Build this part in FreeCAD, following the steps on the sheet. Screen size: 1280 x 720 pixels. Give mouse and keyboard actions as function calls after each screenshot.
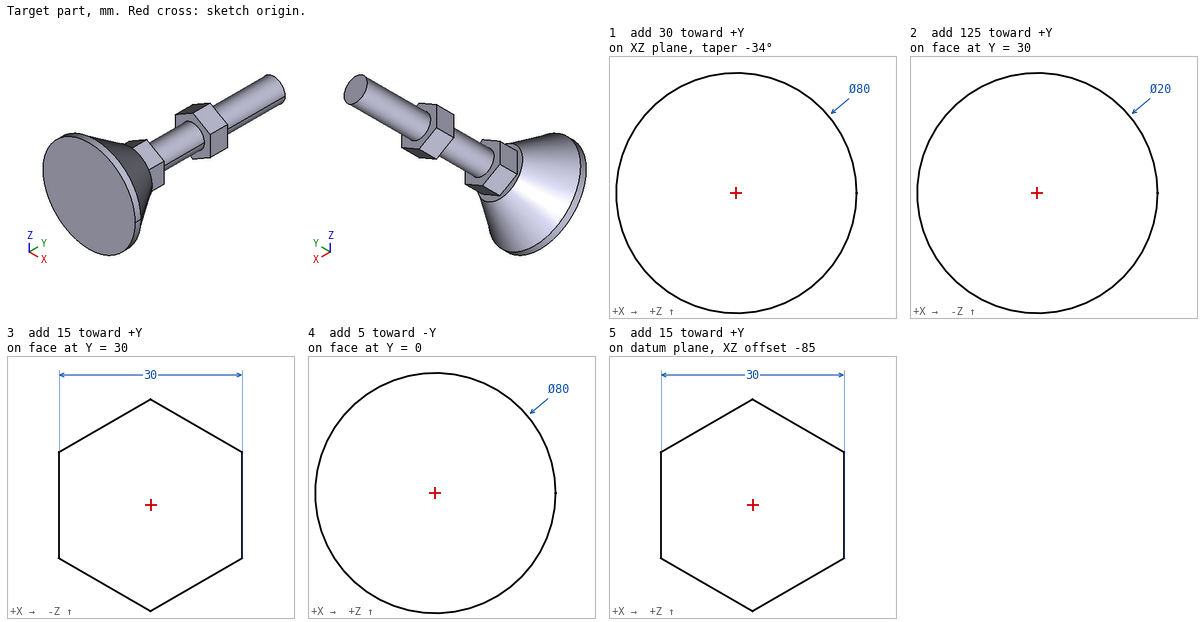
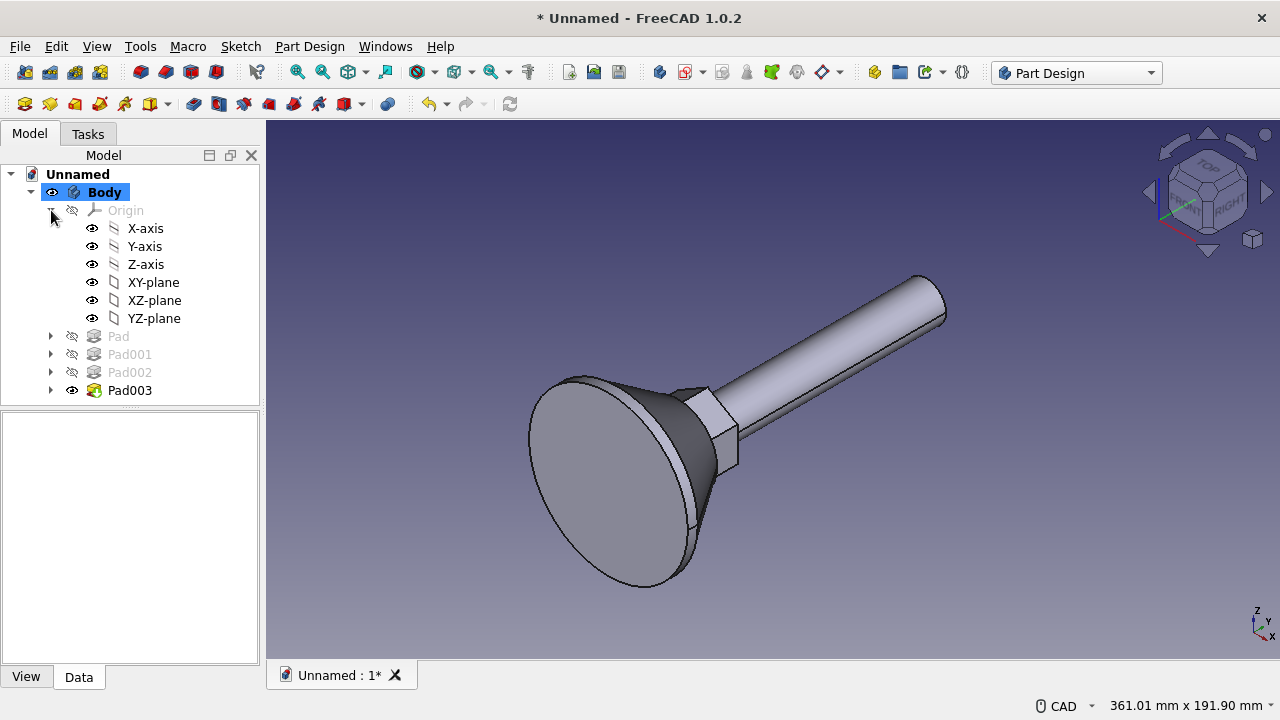
click(137, 300)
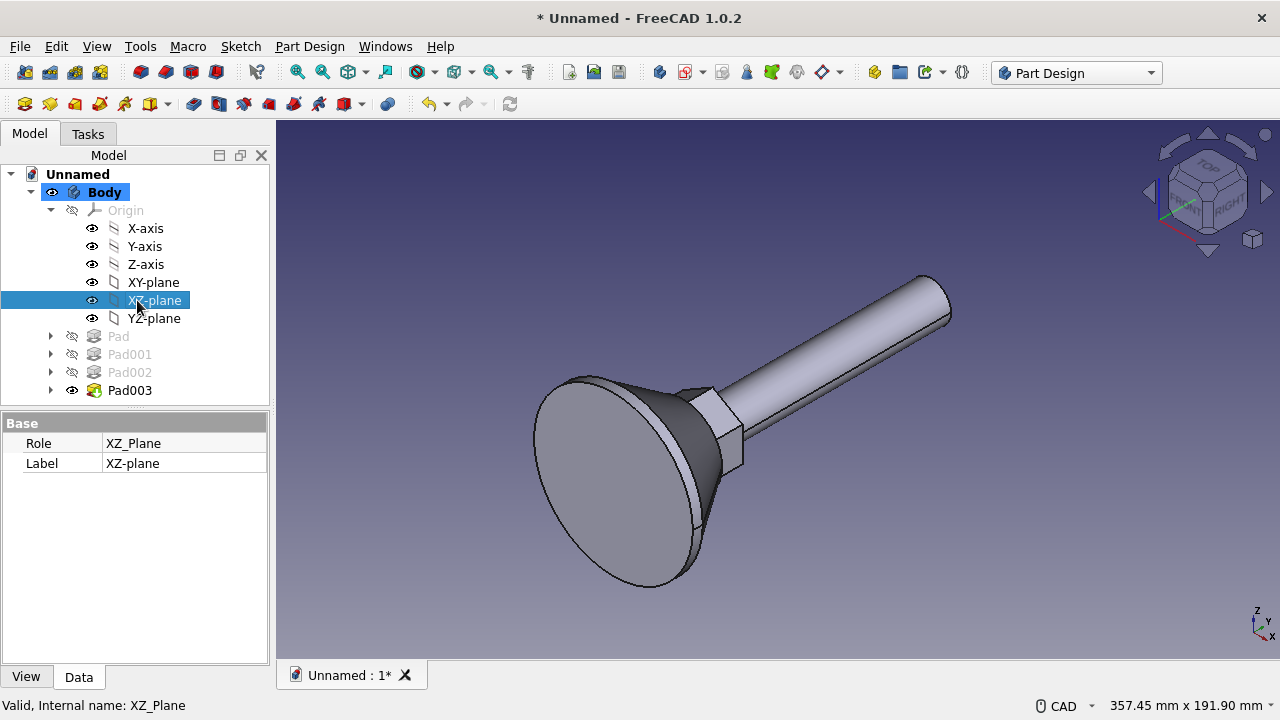
click(822, 72)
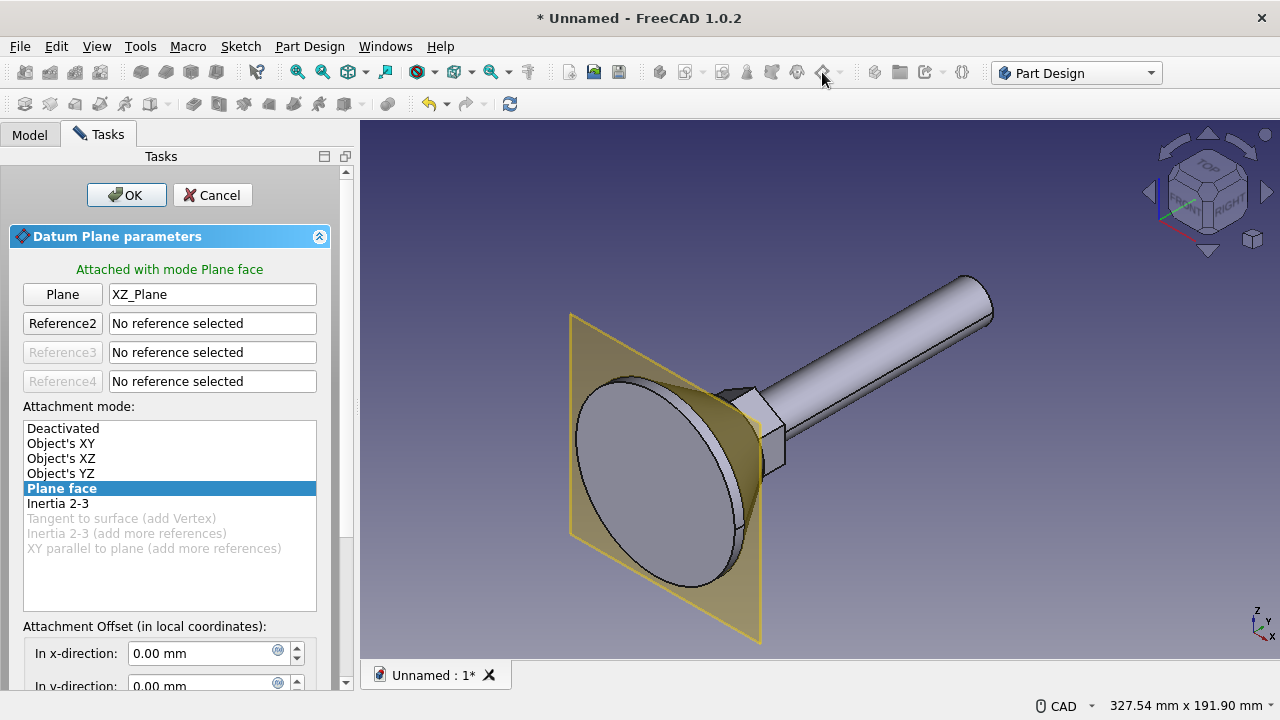
scroll(346, 428, down, 2)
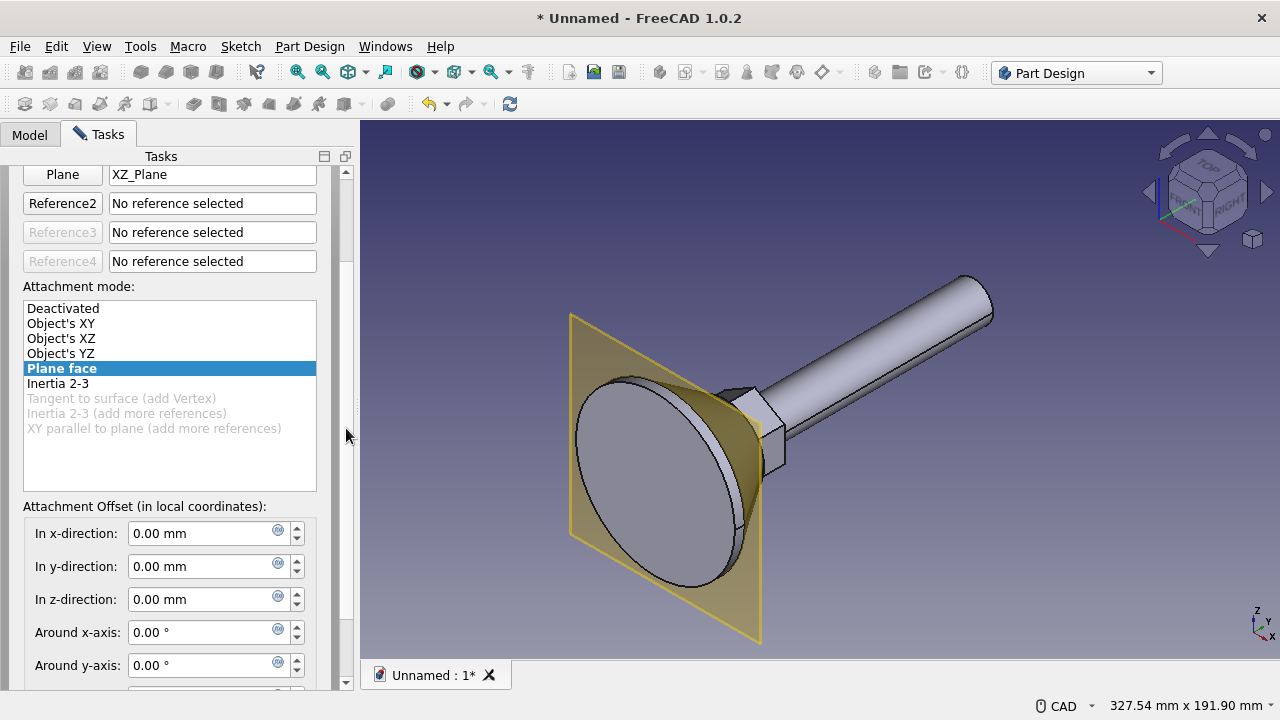
triple_click(210, 600)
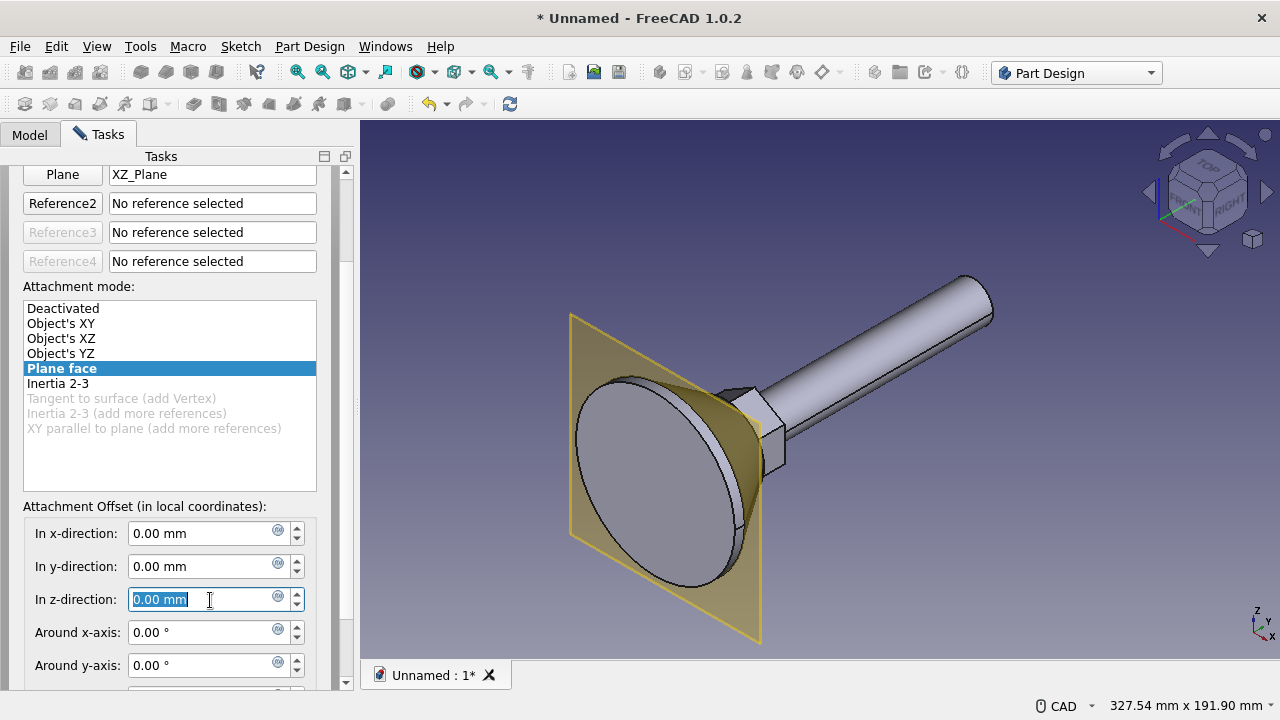
text(-85)
key(Tab)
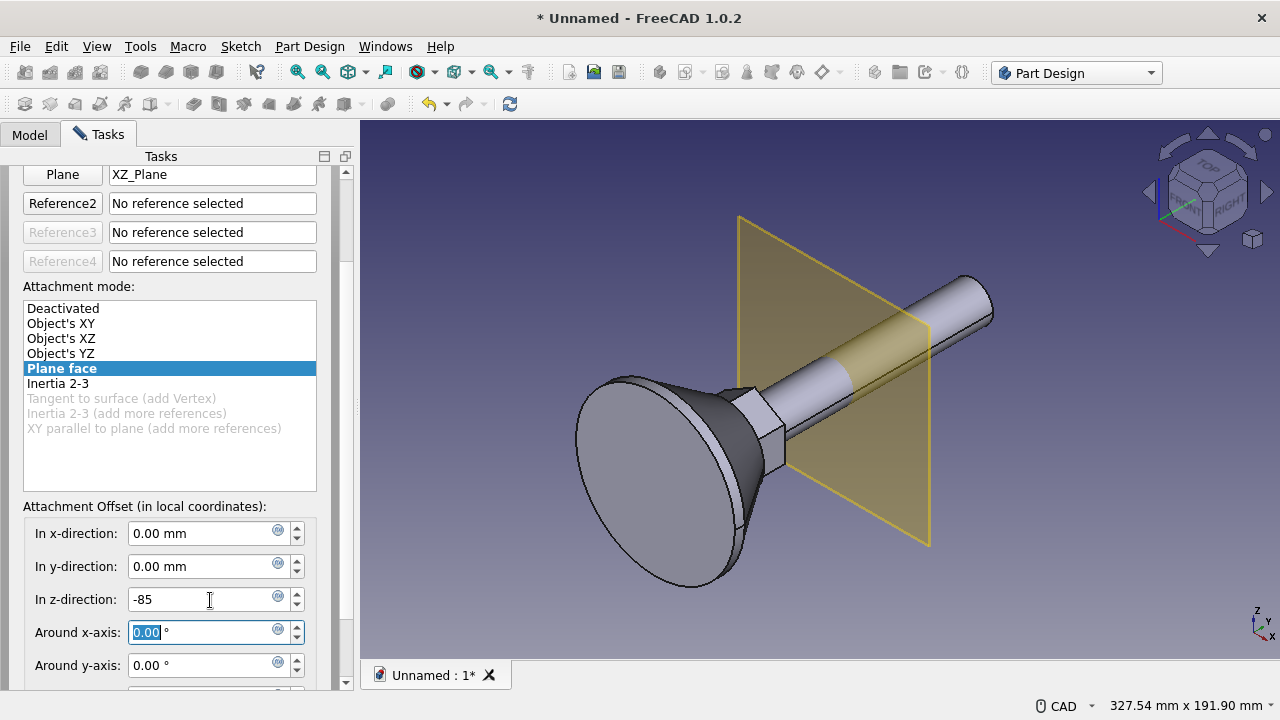
scroll(346, 428, up, 3)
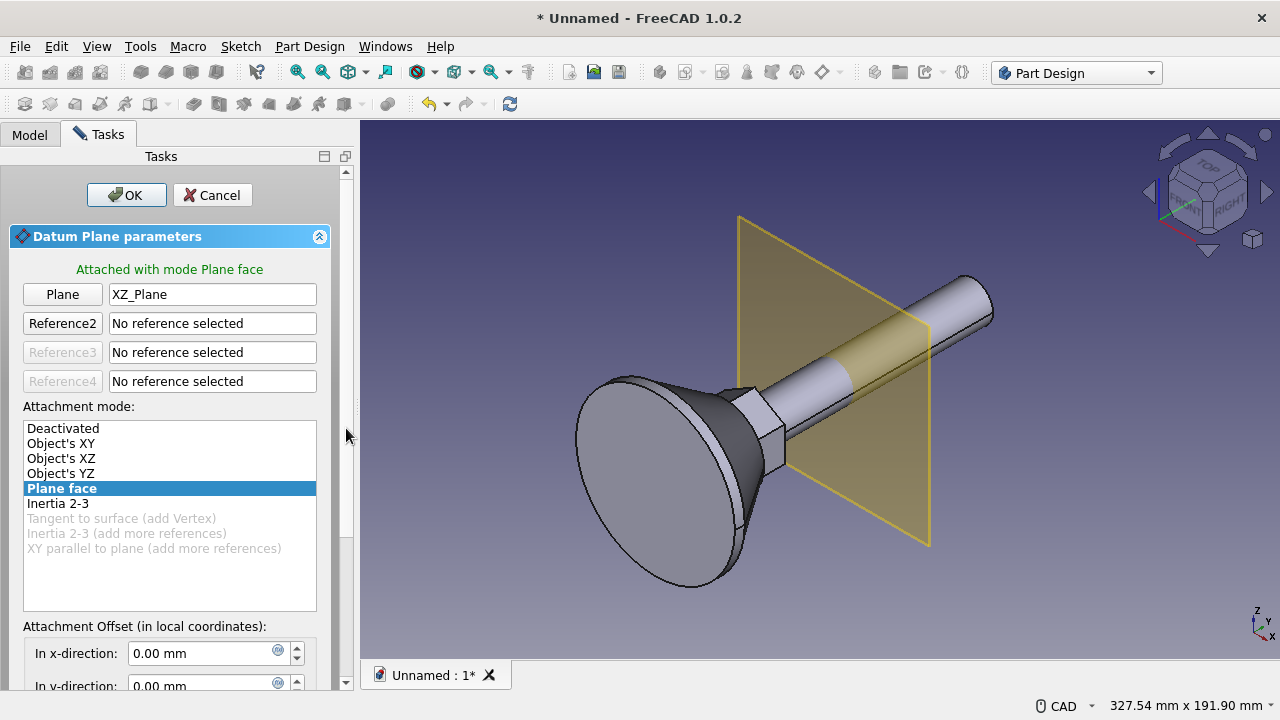
click(127, 195)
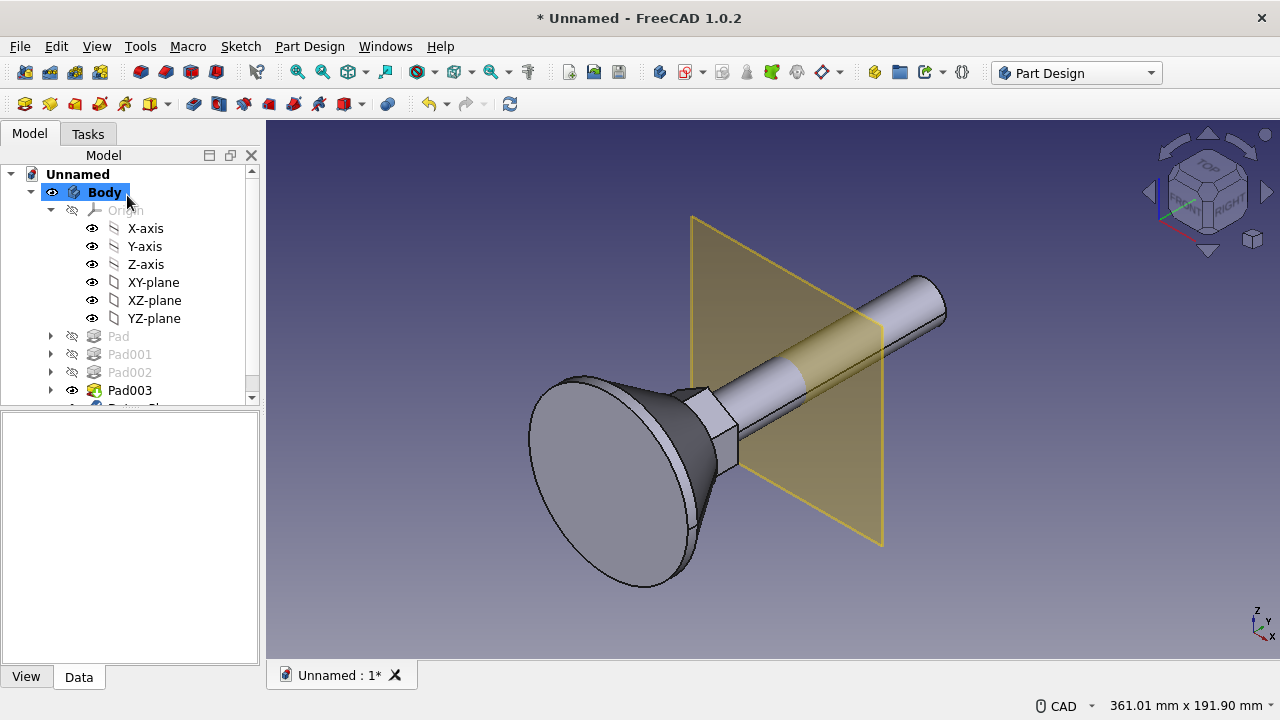
scroll(101, 278, down, 3)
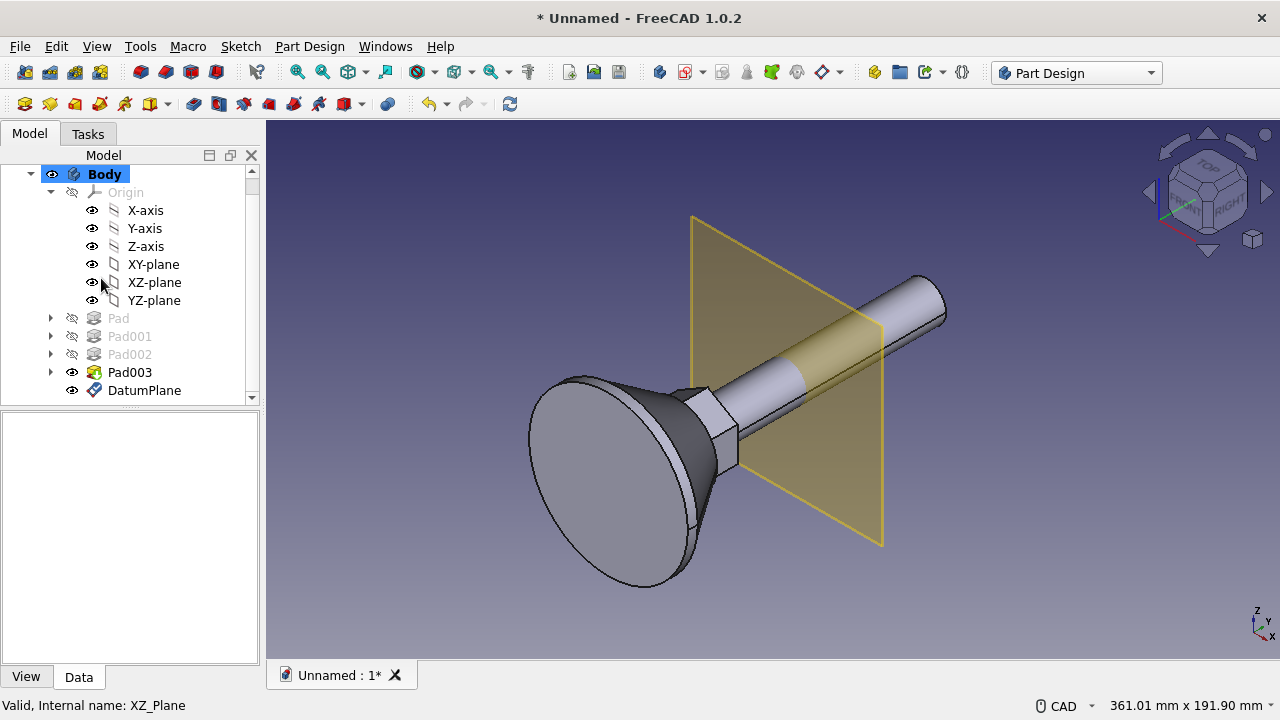
click(117, 390)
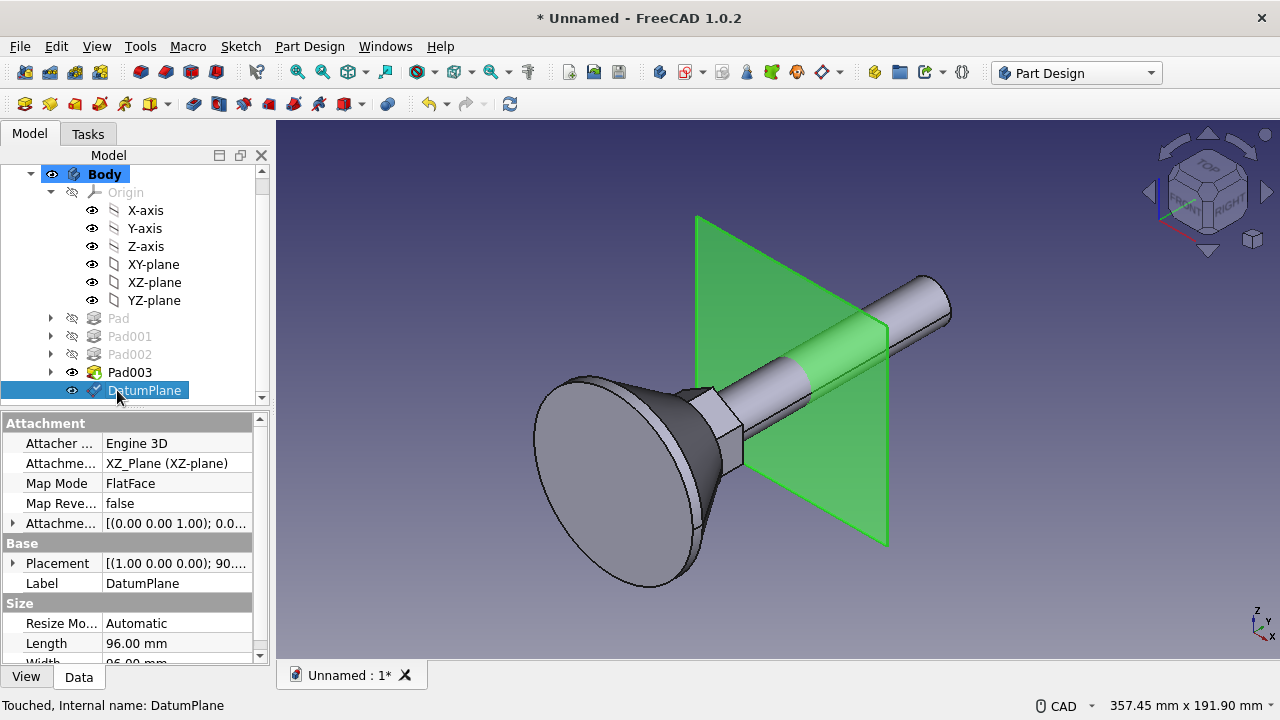
click(684, 72)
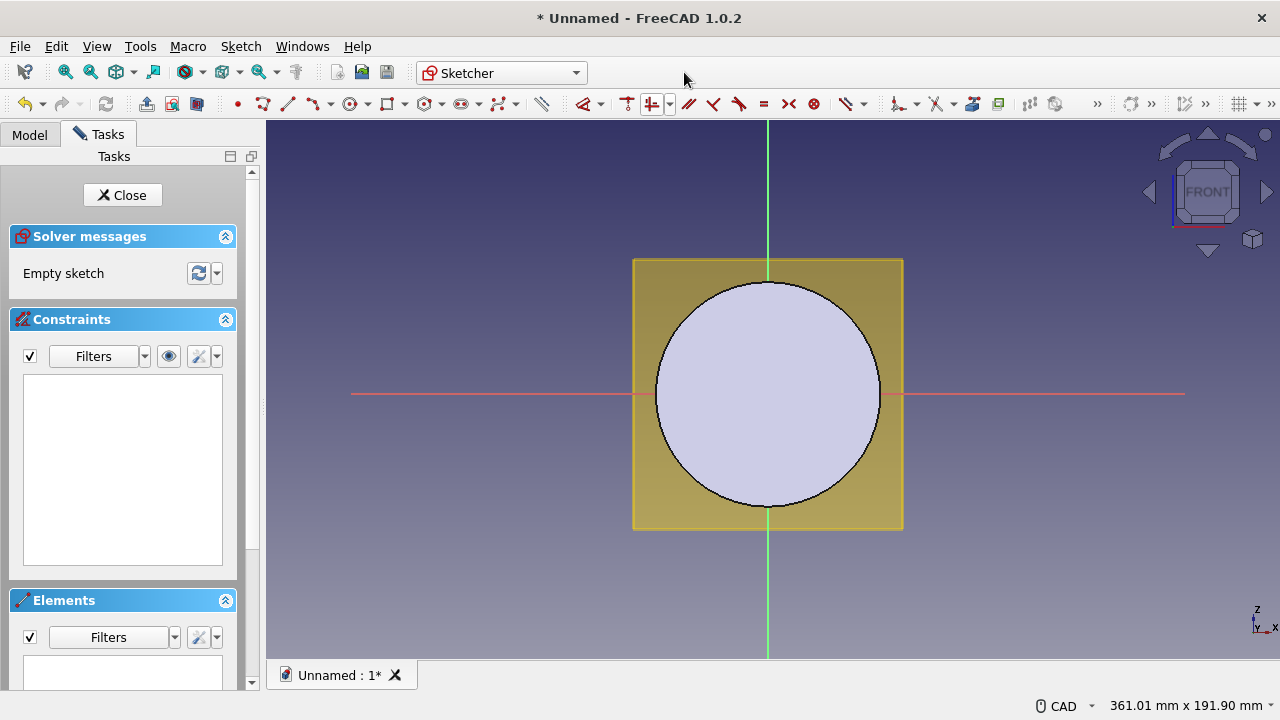
click(197, 104)